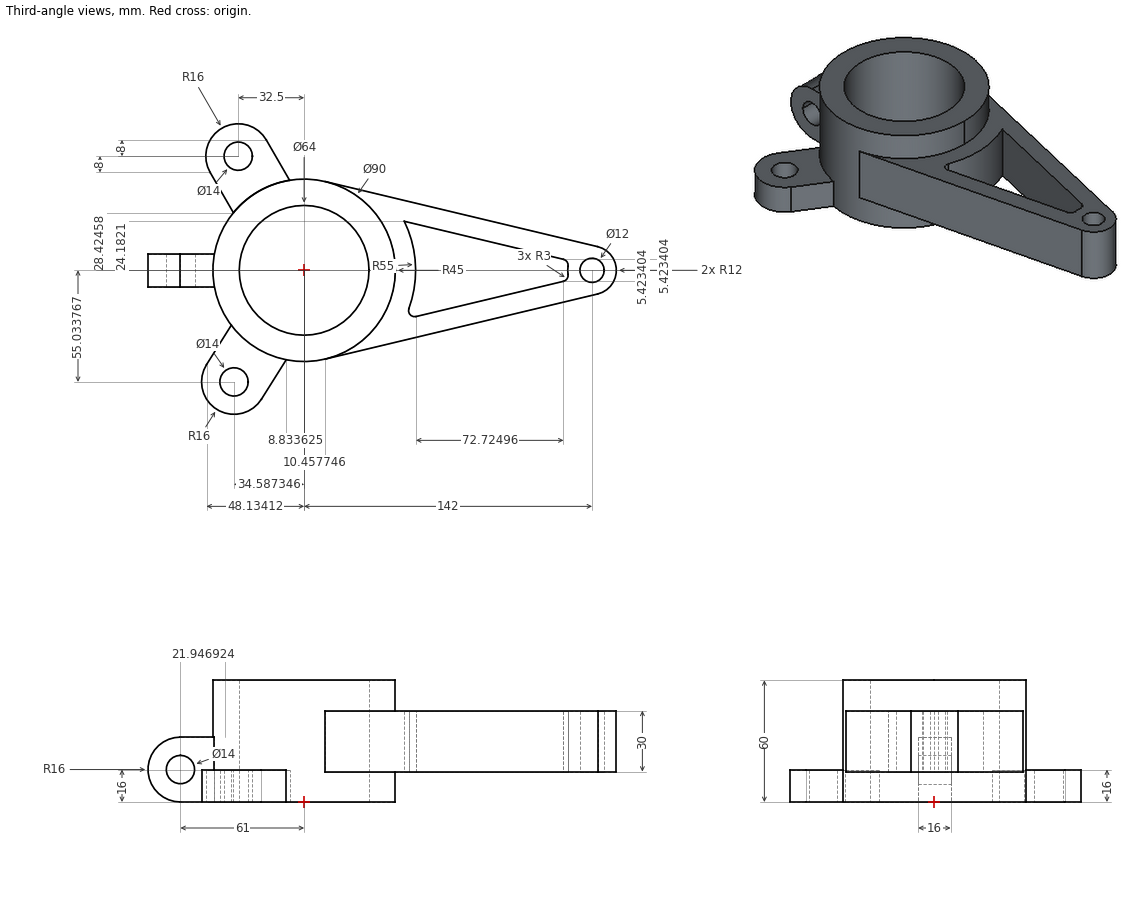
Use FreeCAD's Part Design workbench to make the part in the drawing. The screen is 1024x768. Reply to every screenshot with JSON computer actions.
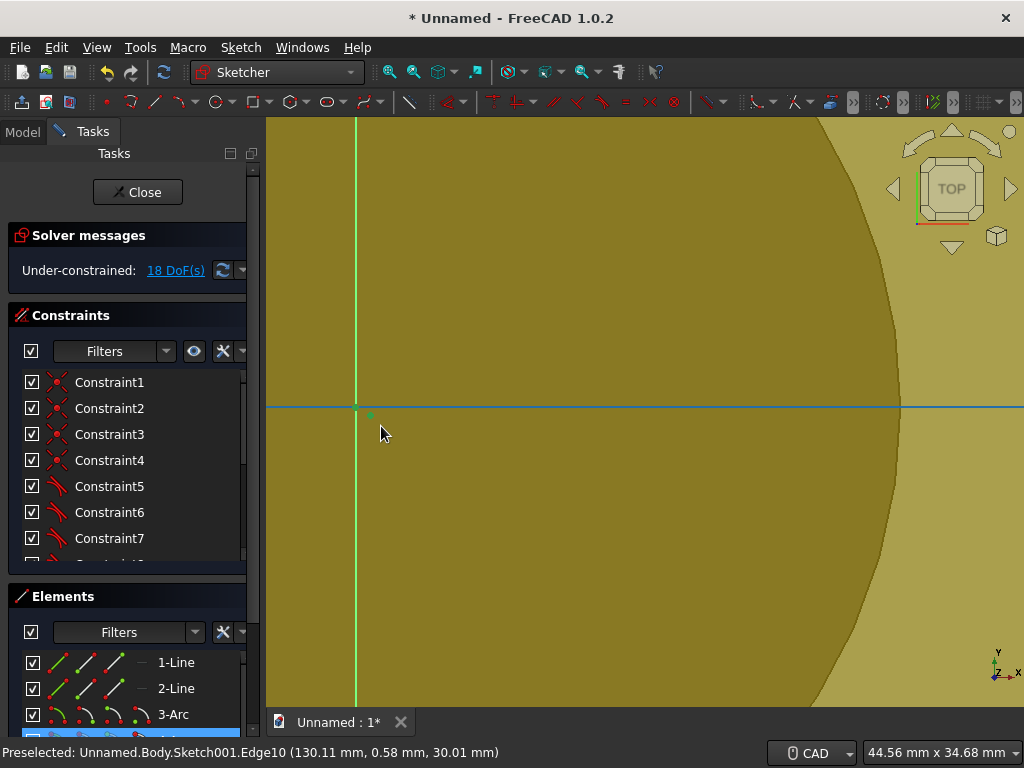
{"action": "left_click", "coordinate": [494, 102]}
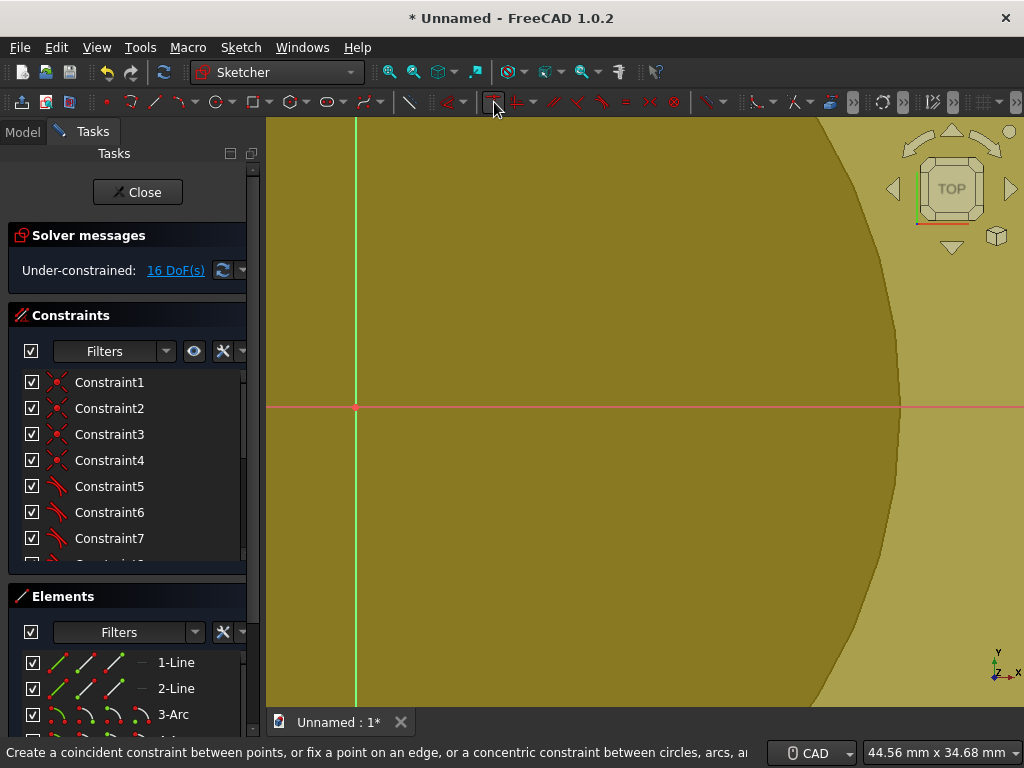
{"action": "scroll", "coordinate": [361, 413], "scroll_direction": "down", "scroll_amount": 9}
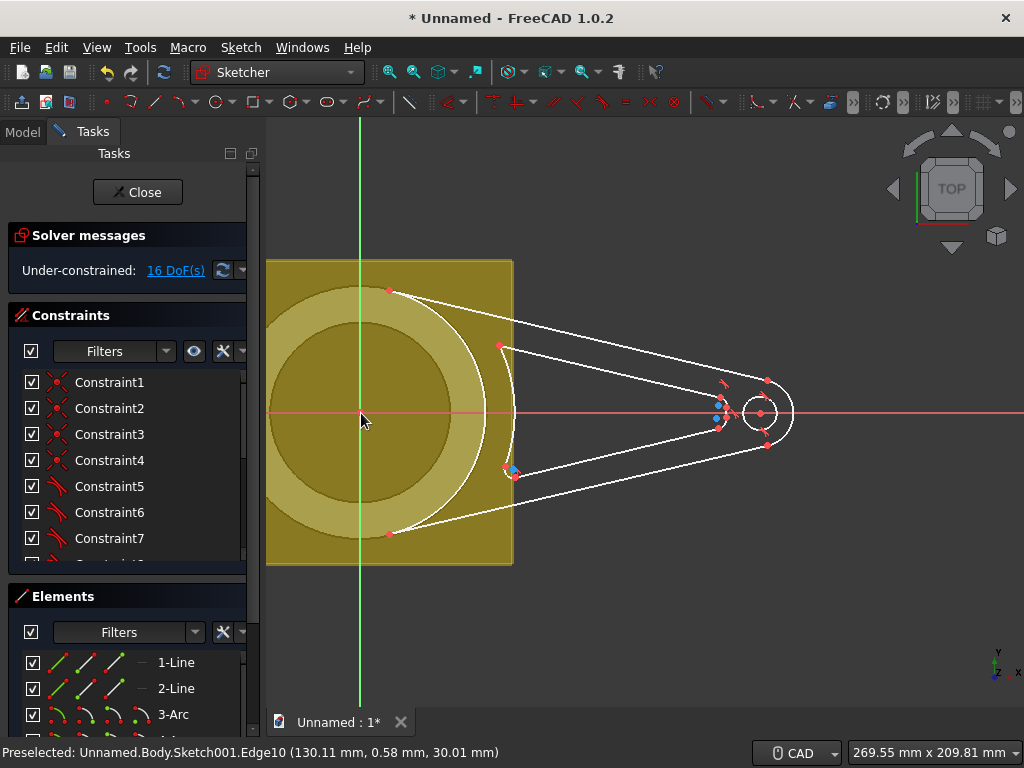
{"action": "scroll", "coordinate": [505, 472], "scroll_direction": "up", "scroll_amount": 5}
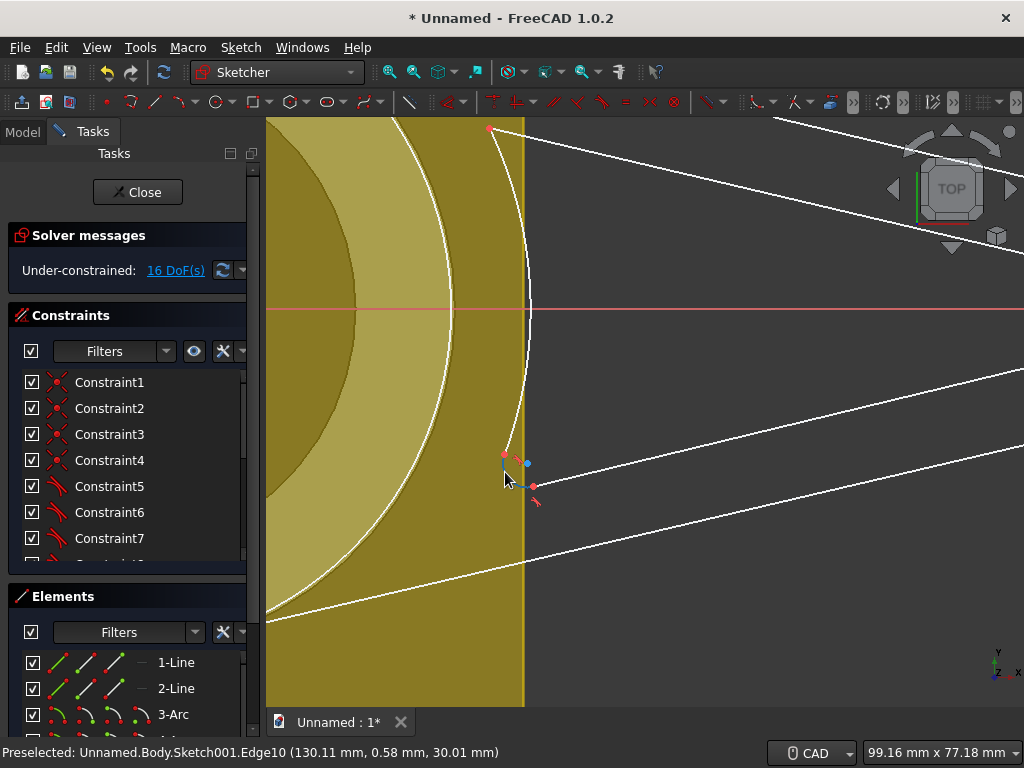
{"action": "left_click", "coordinate": [504, 470]}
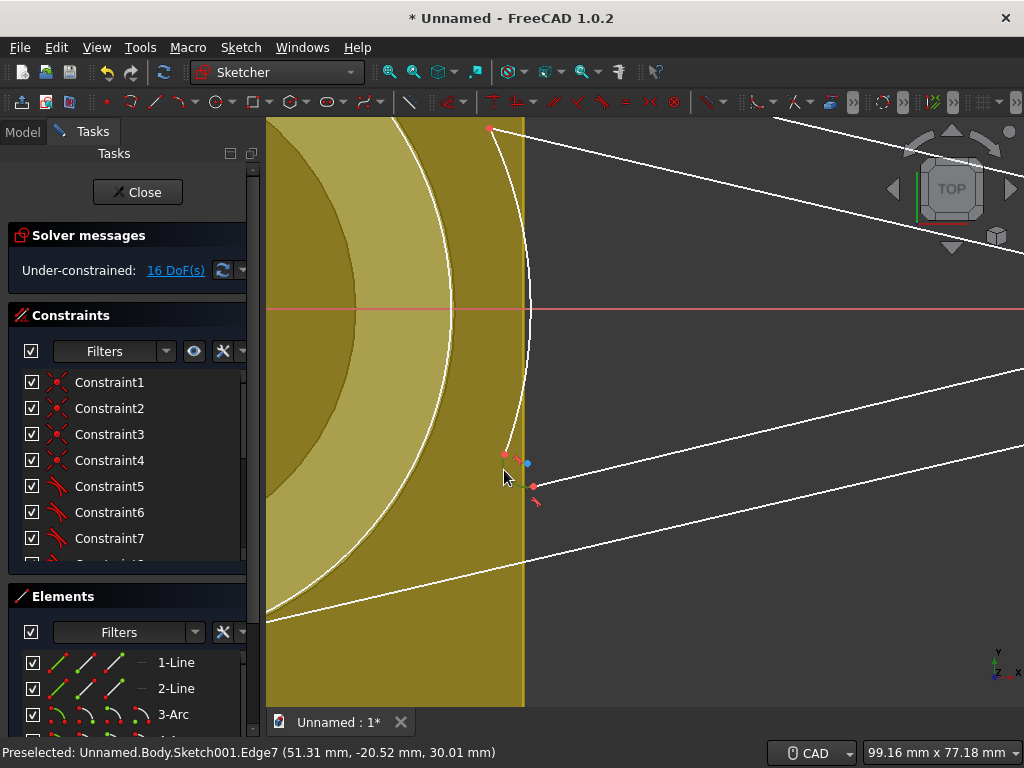
{"action": "scroll", "coordinate": [505, 472], "scroll_direction": "down", "scroll_amount": 5}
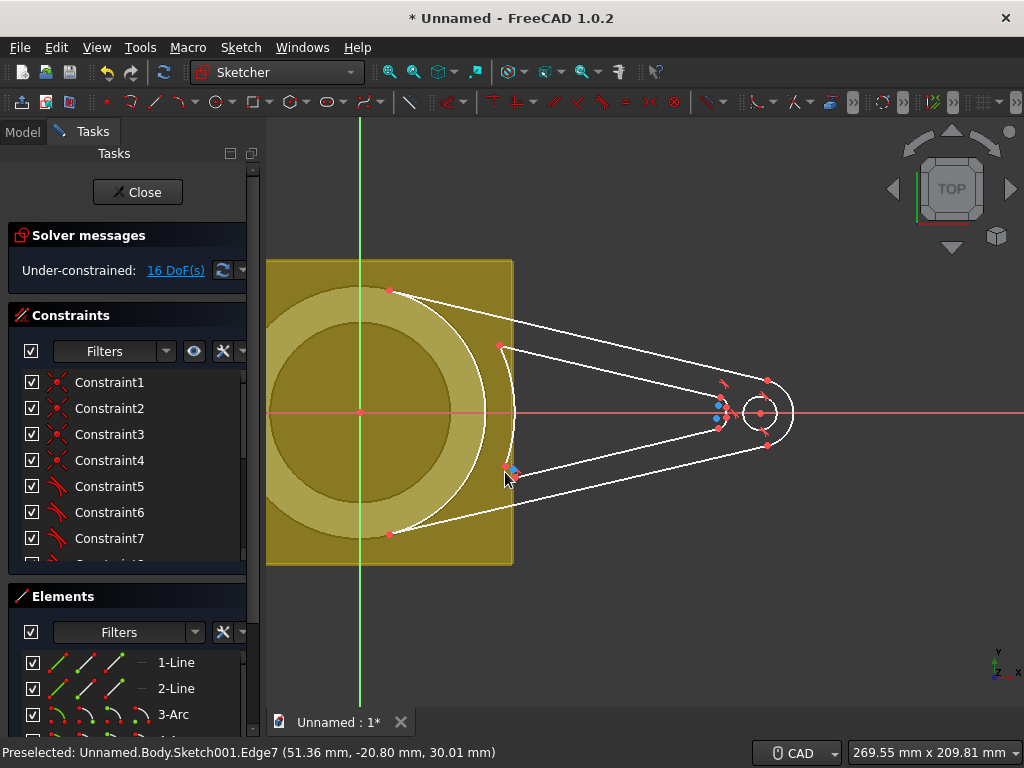
{"action": "scroll", "coordinate": [727, 403], "scroll_direction": "up", "scroll_amount": 7}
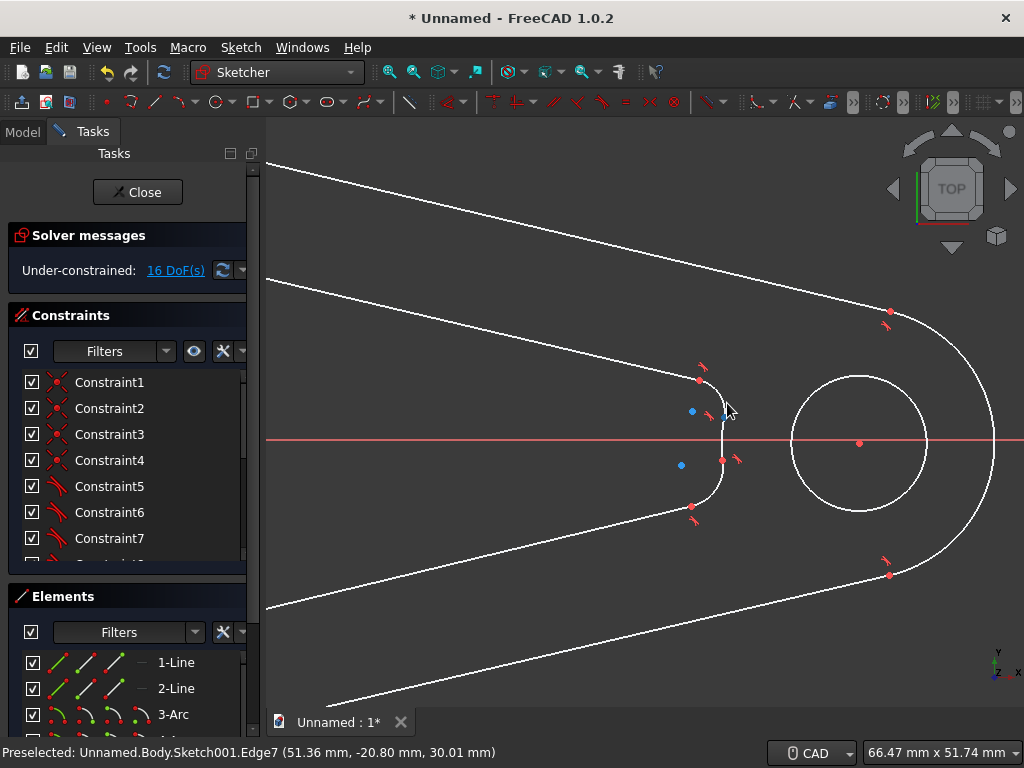
{"action": "left_click", "coordinate": [724, 403]}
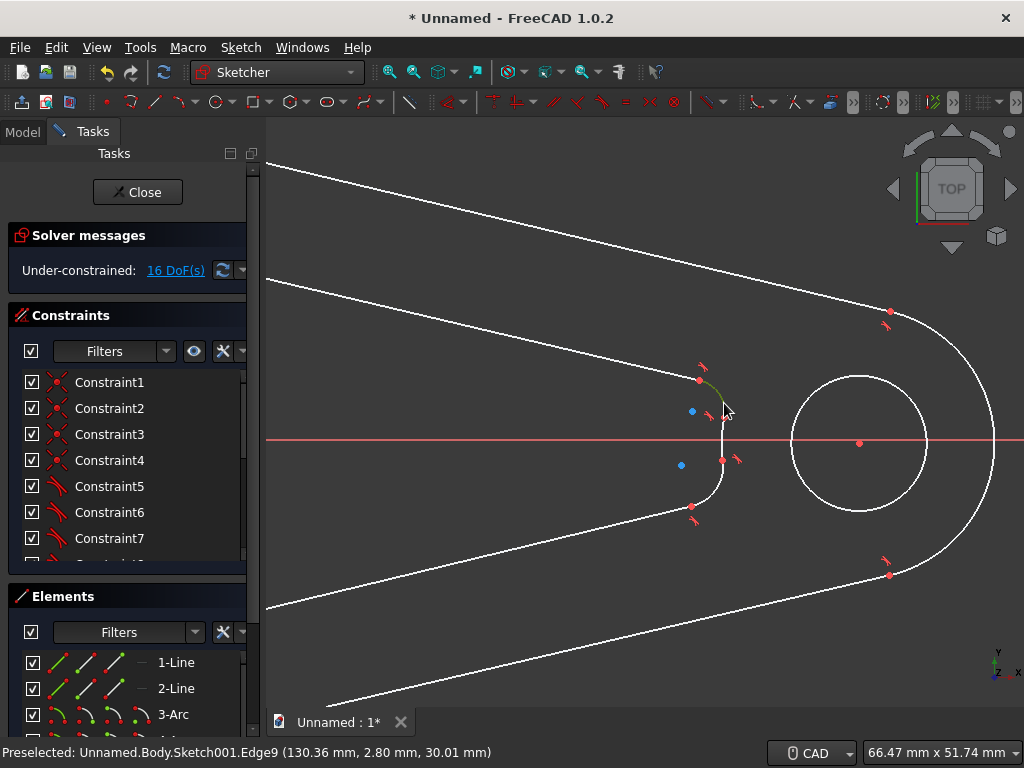
{"action": "left_click", "coordinate": [708, 498]}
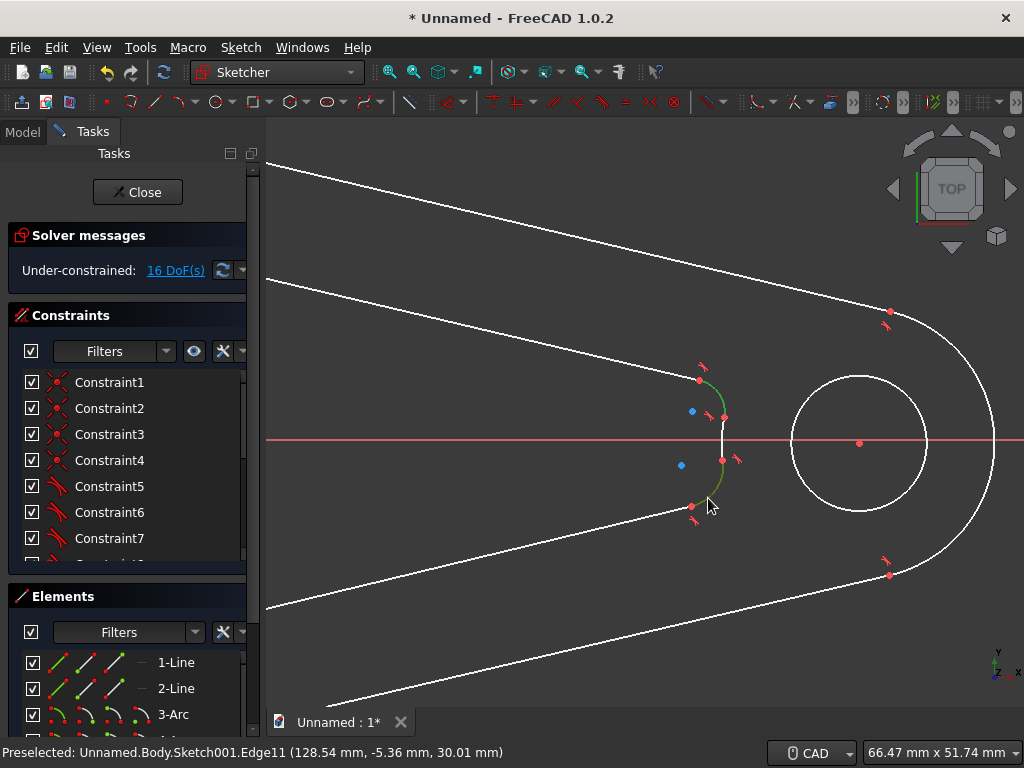
{"action": "key", "text": "e"}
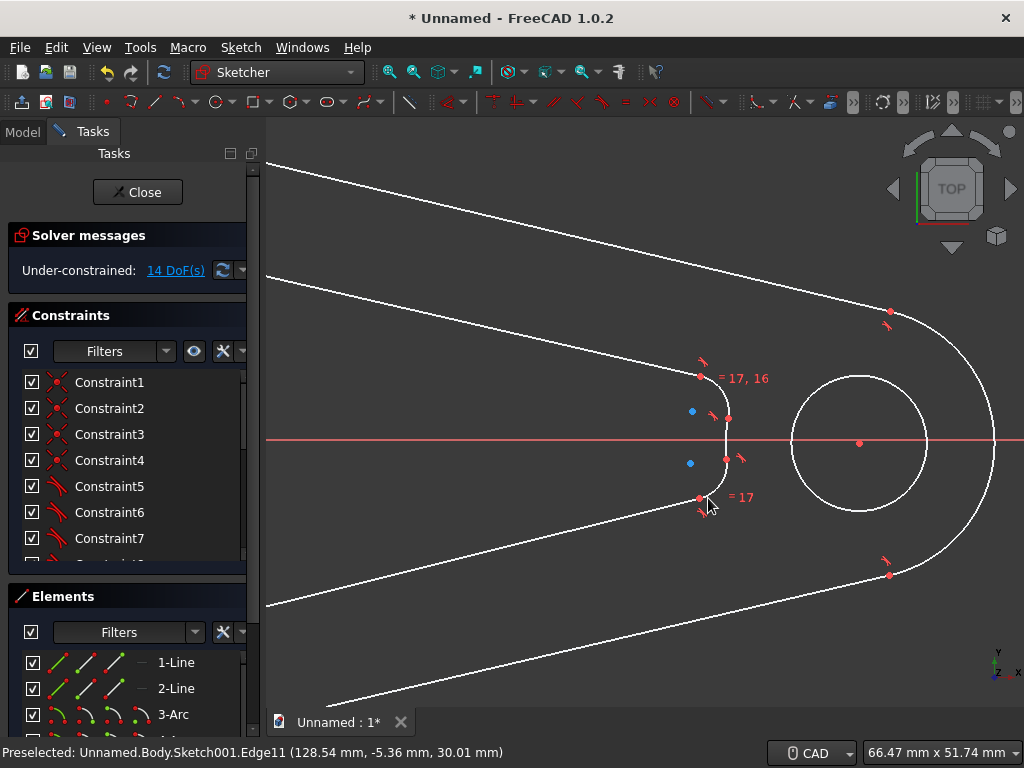
{"action": "scroll", "coordinate": [727, 403], "scroll_direction": "down", "scroll_amount": 7}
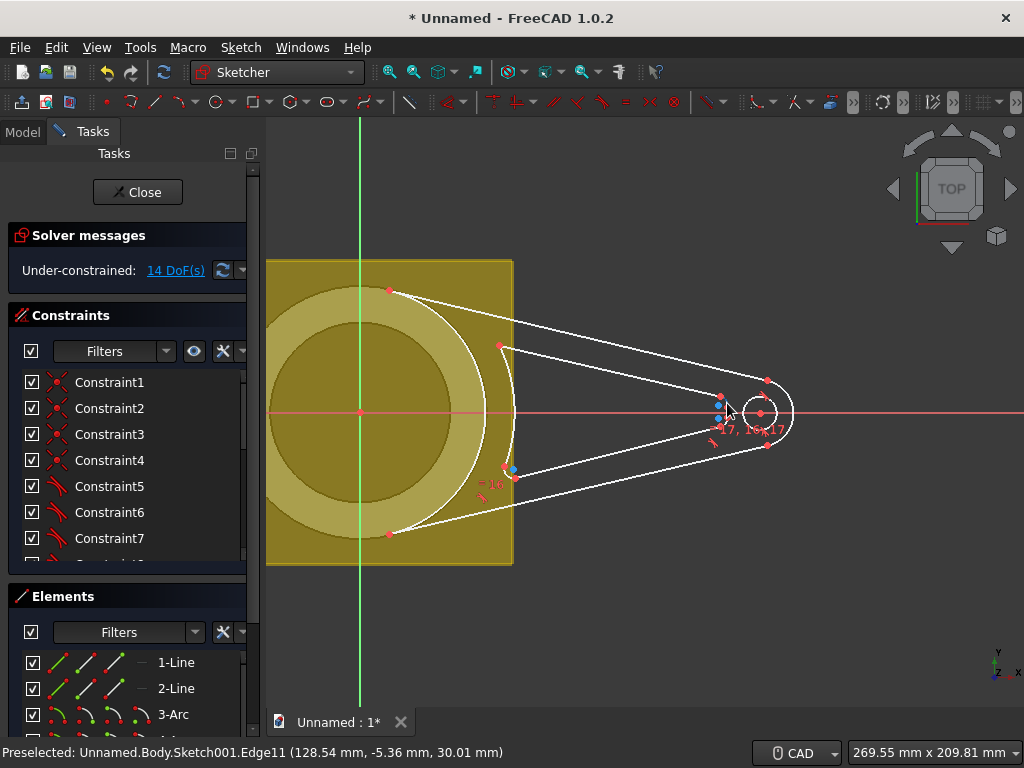
{"action": "left_click", "coordinate": [789, 430]}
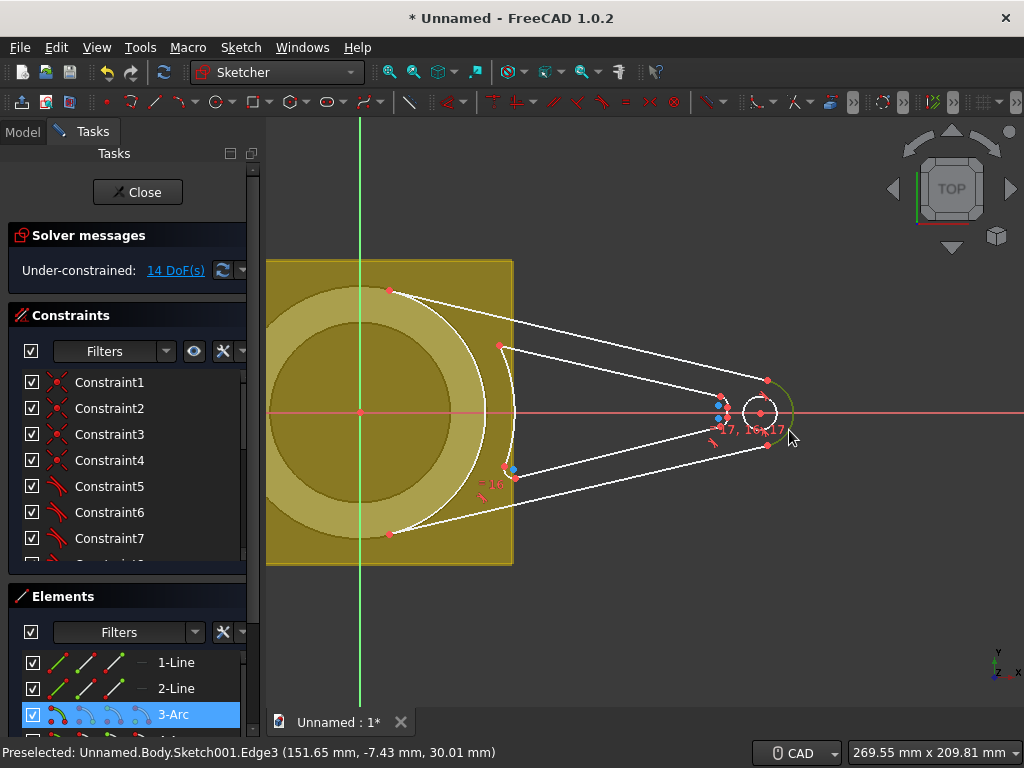
{"action": "scroll", "coordinate": [727, 412], "scroll_direction": "up", "scroll_amount": 6}